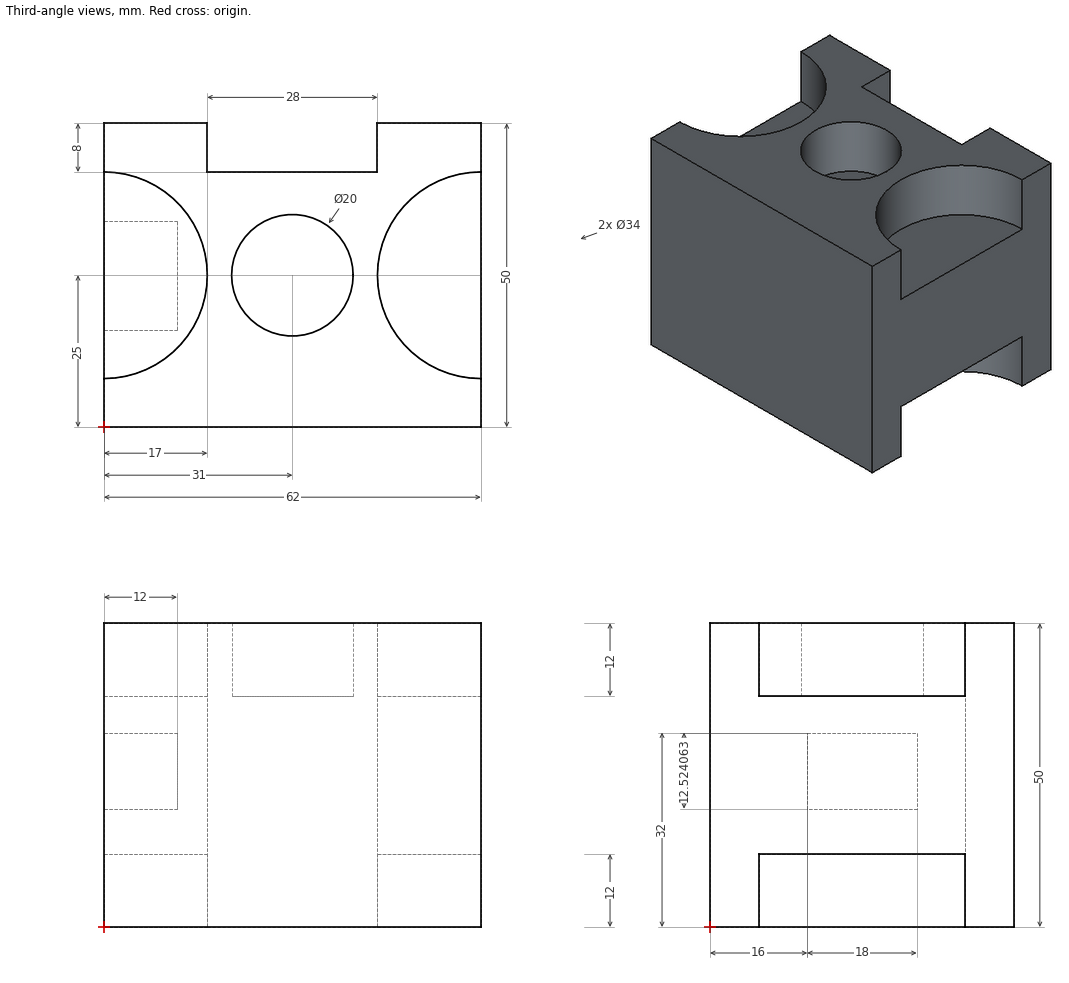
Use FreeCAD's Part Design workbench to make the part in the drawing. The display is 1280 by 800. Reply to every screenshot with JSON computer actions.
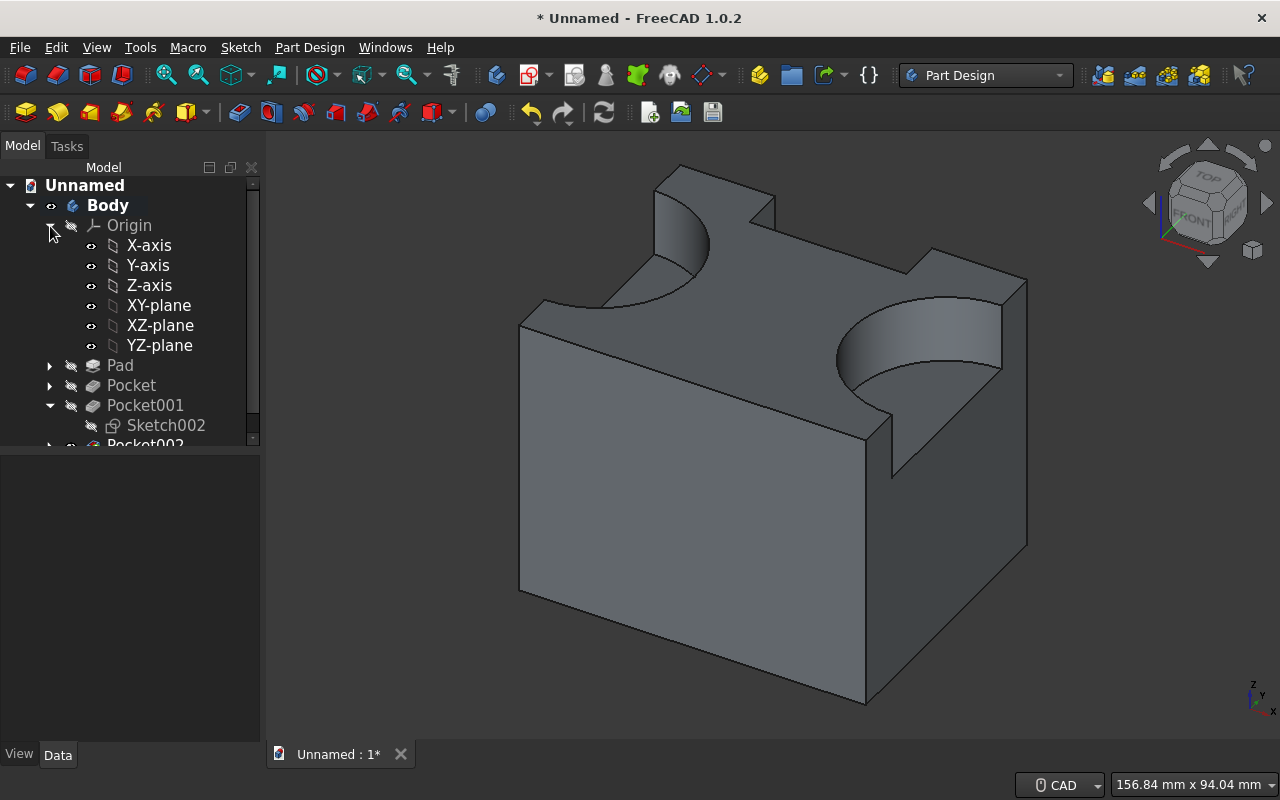
{"action": "left_click", "coordinate": [136, 306]}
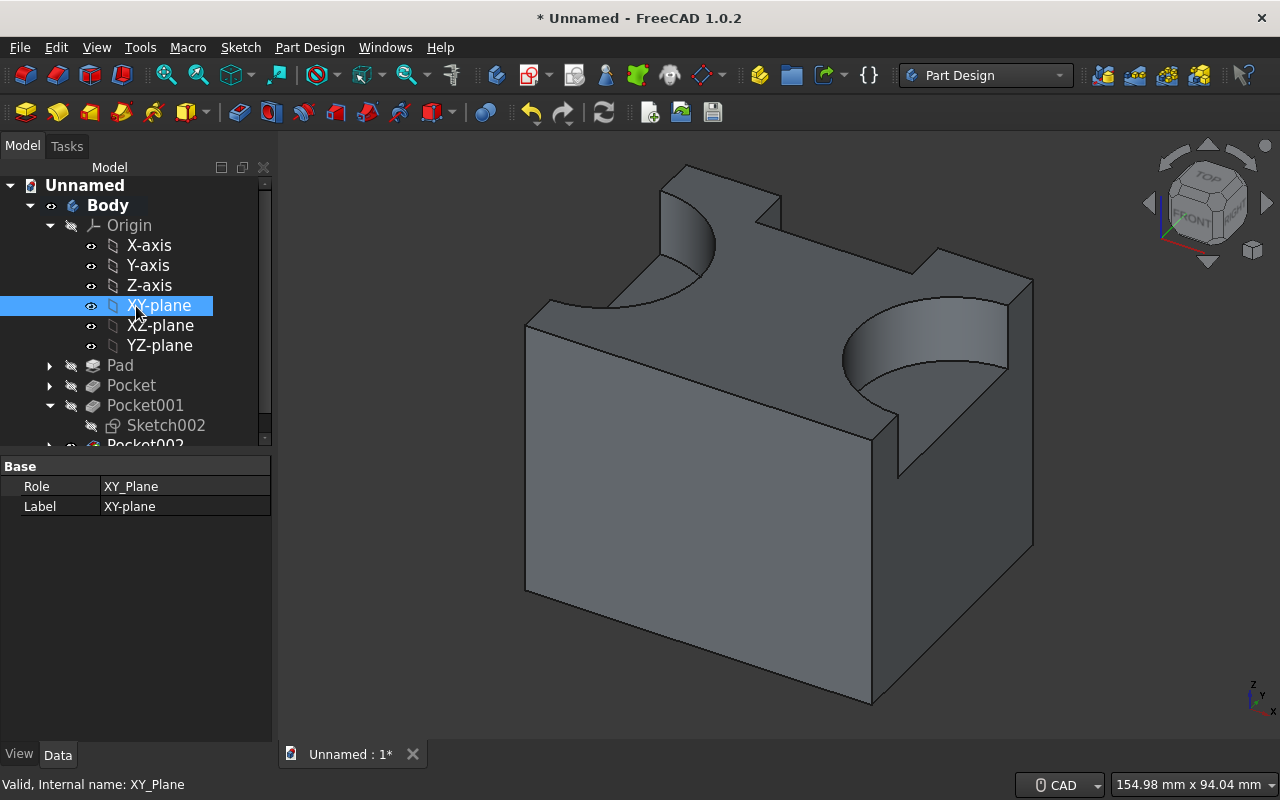
{"action": "left_click", "coordinate": [702, 76]}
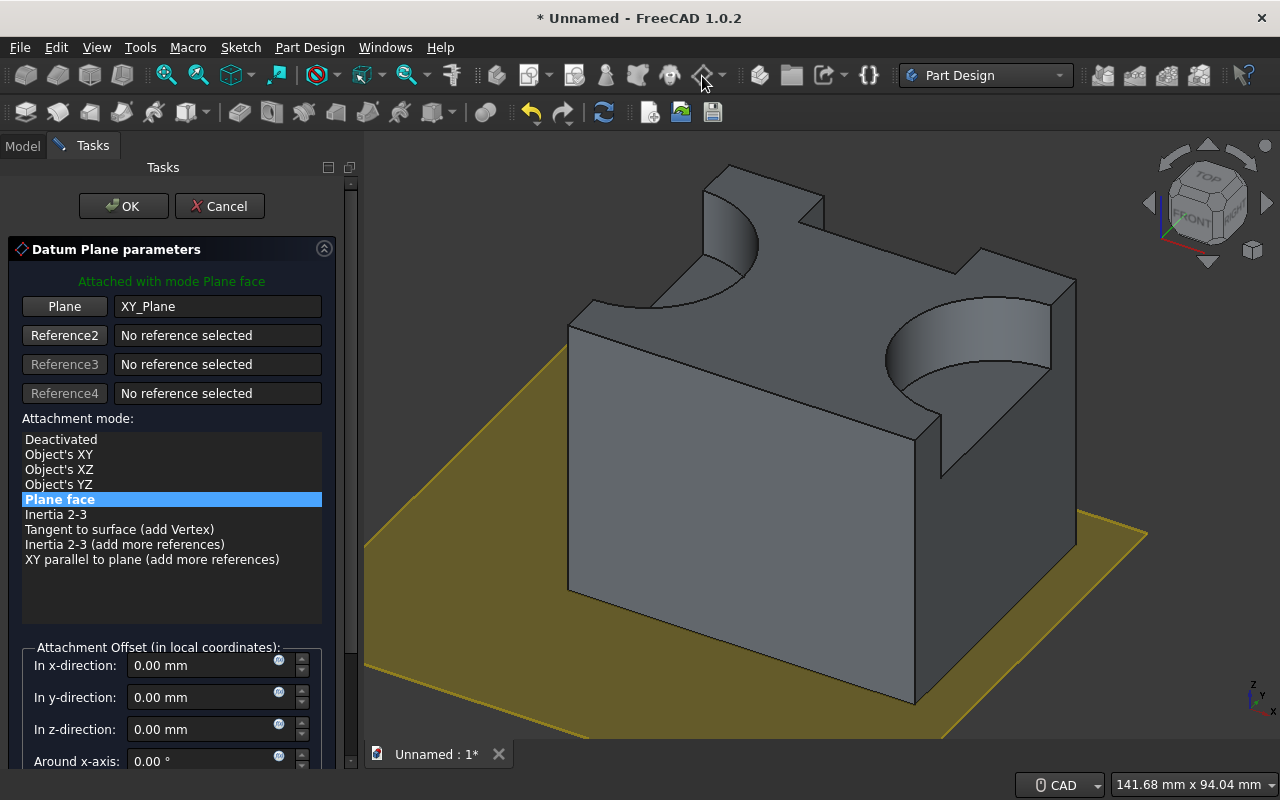
{"action": "triple_click", "coordinate": [210, 729]}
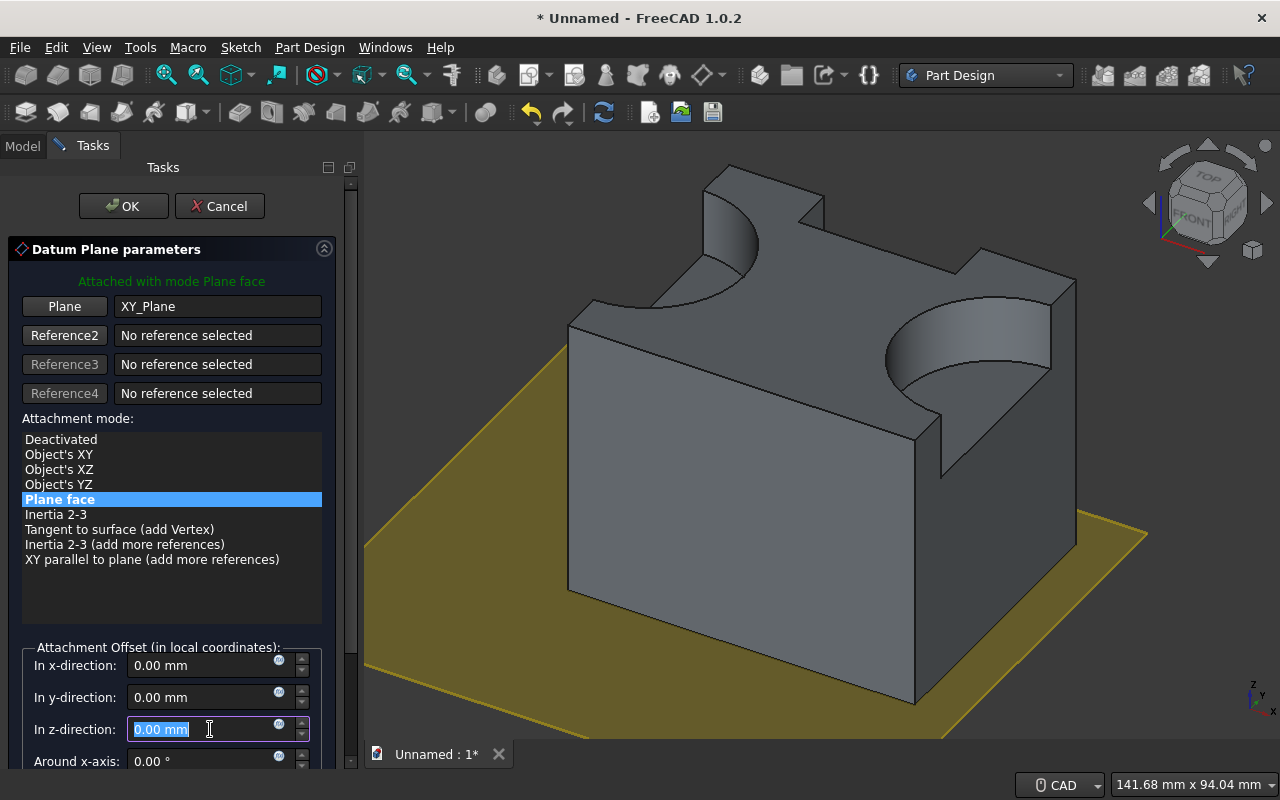
{"action": "type", "text": "12"}
{"action": "key", "text": "Tab"}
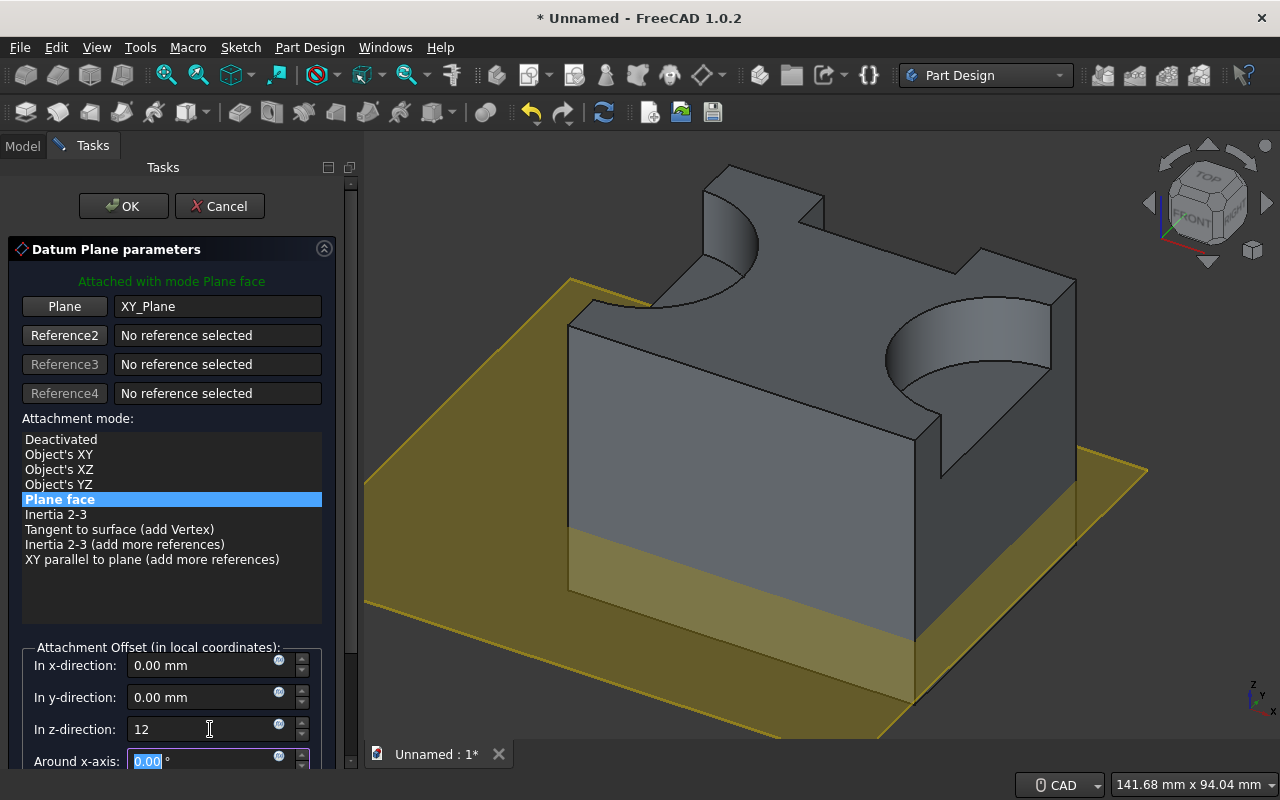
{"action": "left_click", "coordinate": [124, 206]}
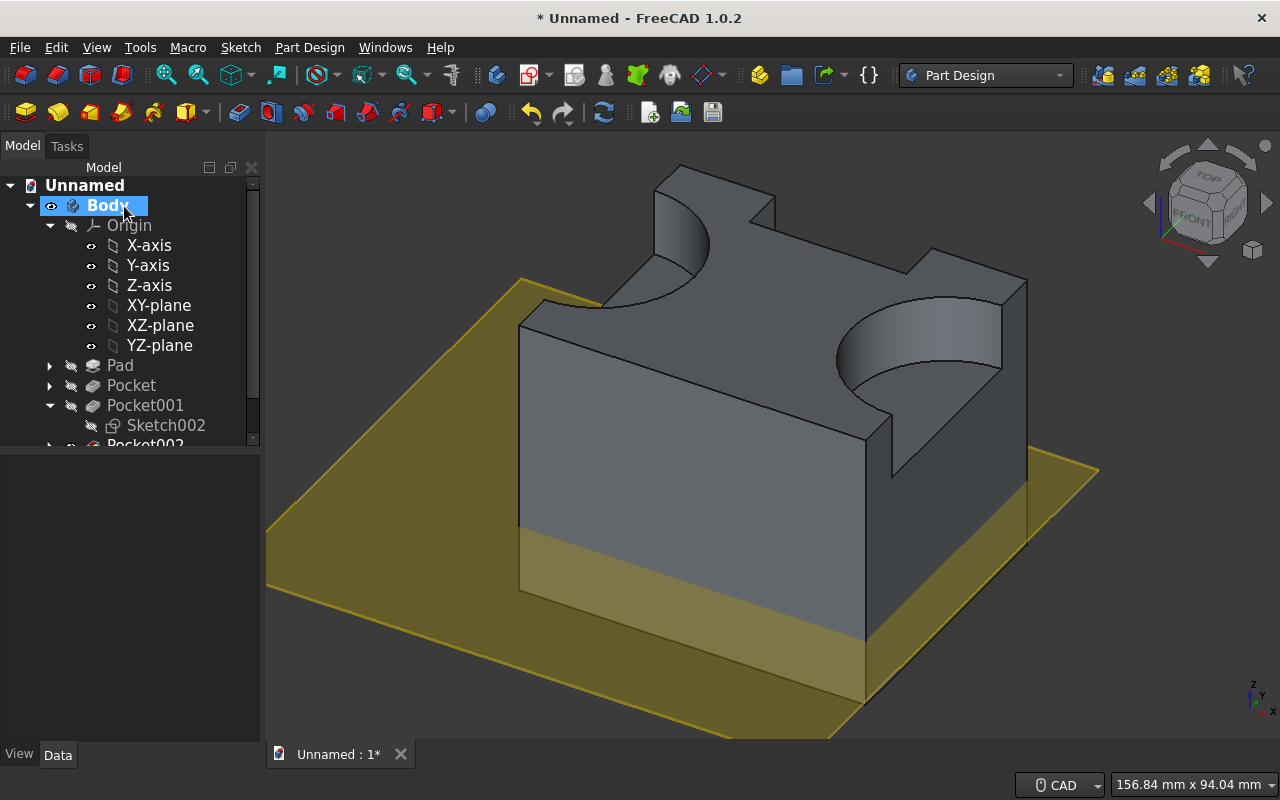
{"action": "scroll", "coordinate": [100, 321], "scroll_direction": "down", "scroll_amount": 3}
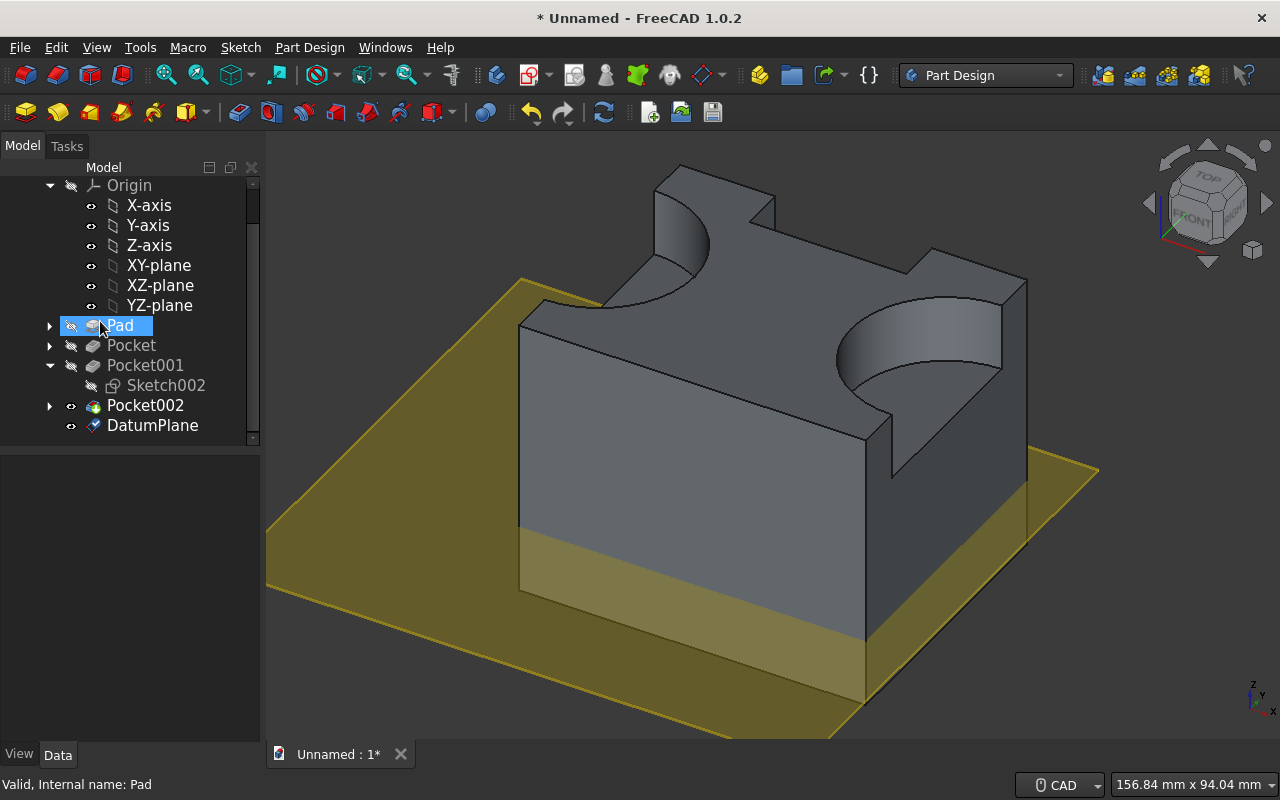
{"action": "left_click", "coordinate": [116, 426]}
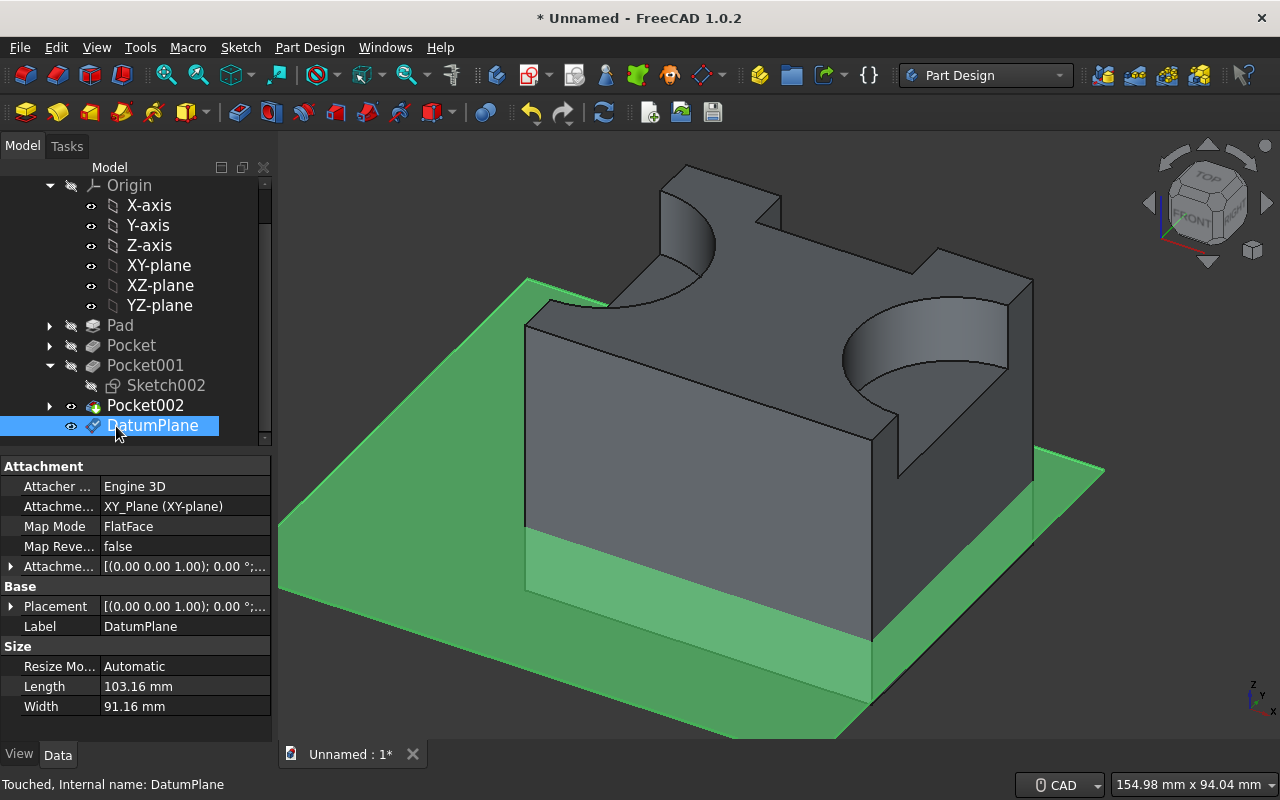
{"action": "left_click", "coordinate": [530, 76]}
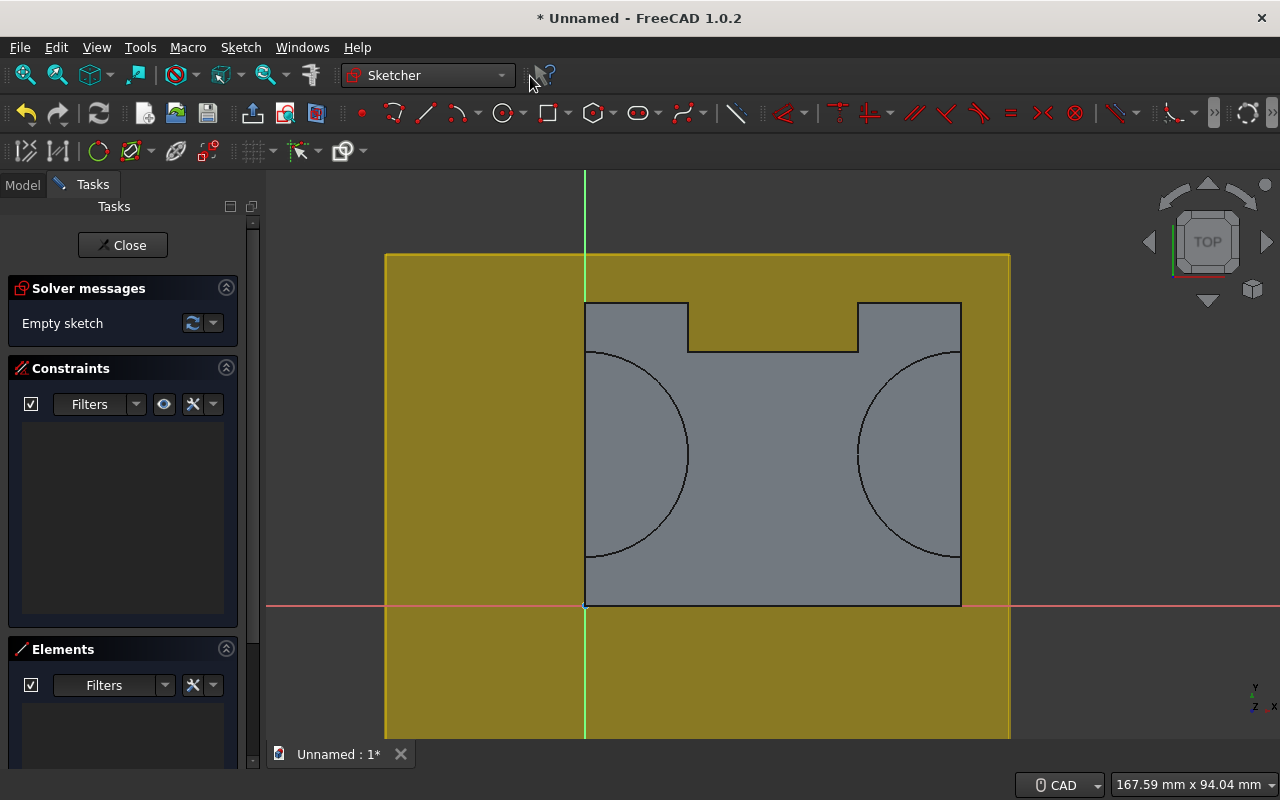
{"action": "left_click", "coordinate": [318, 114]}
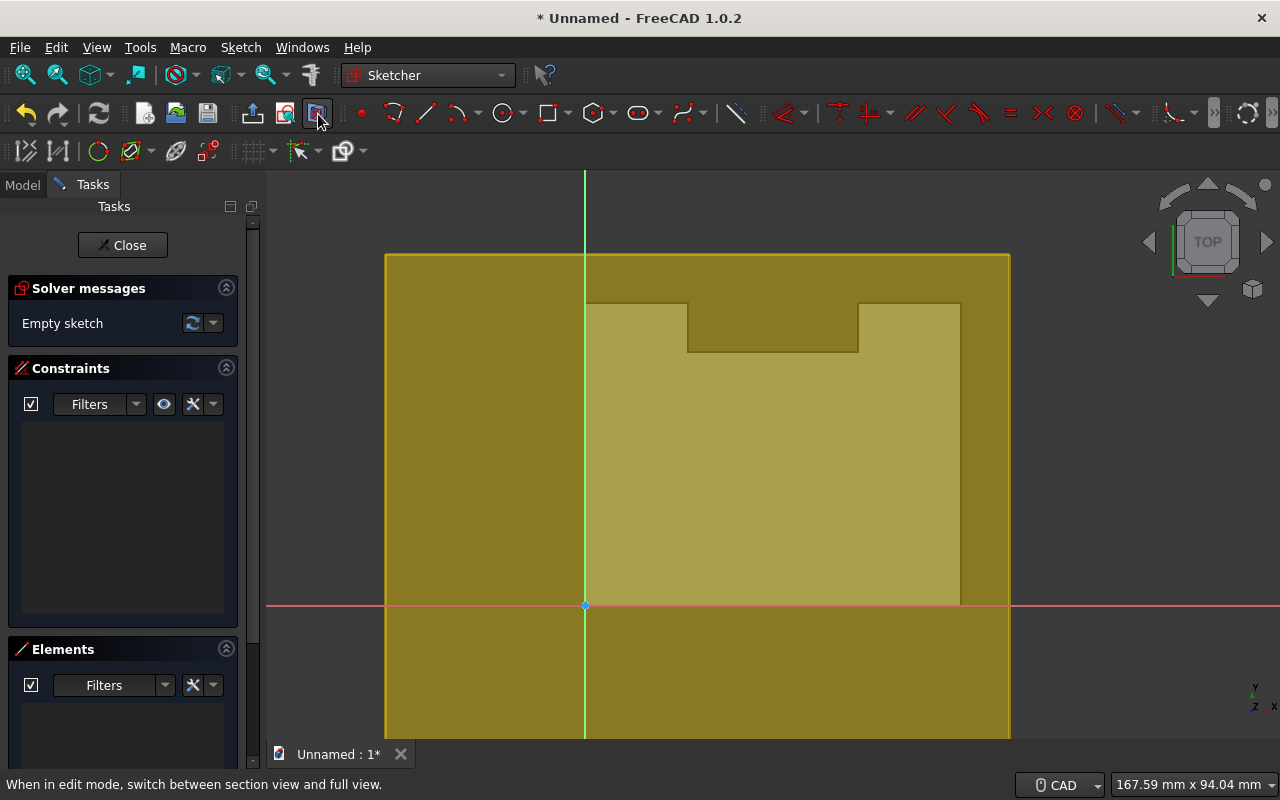
{"action": "left_click", "coordinate": [504, 114]}